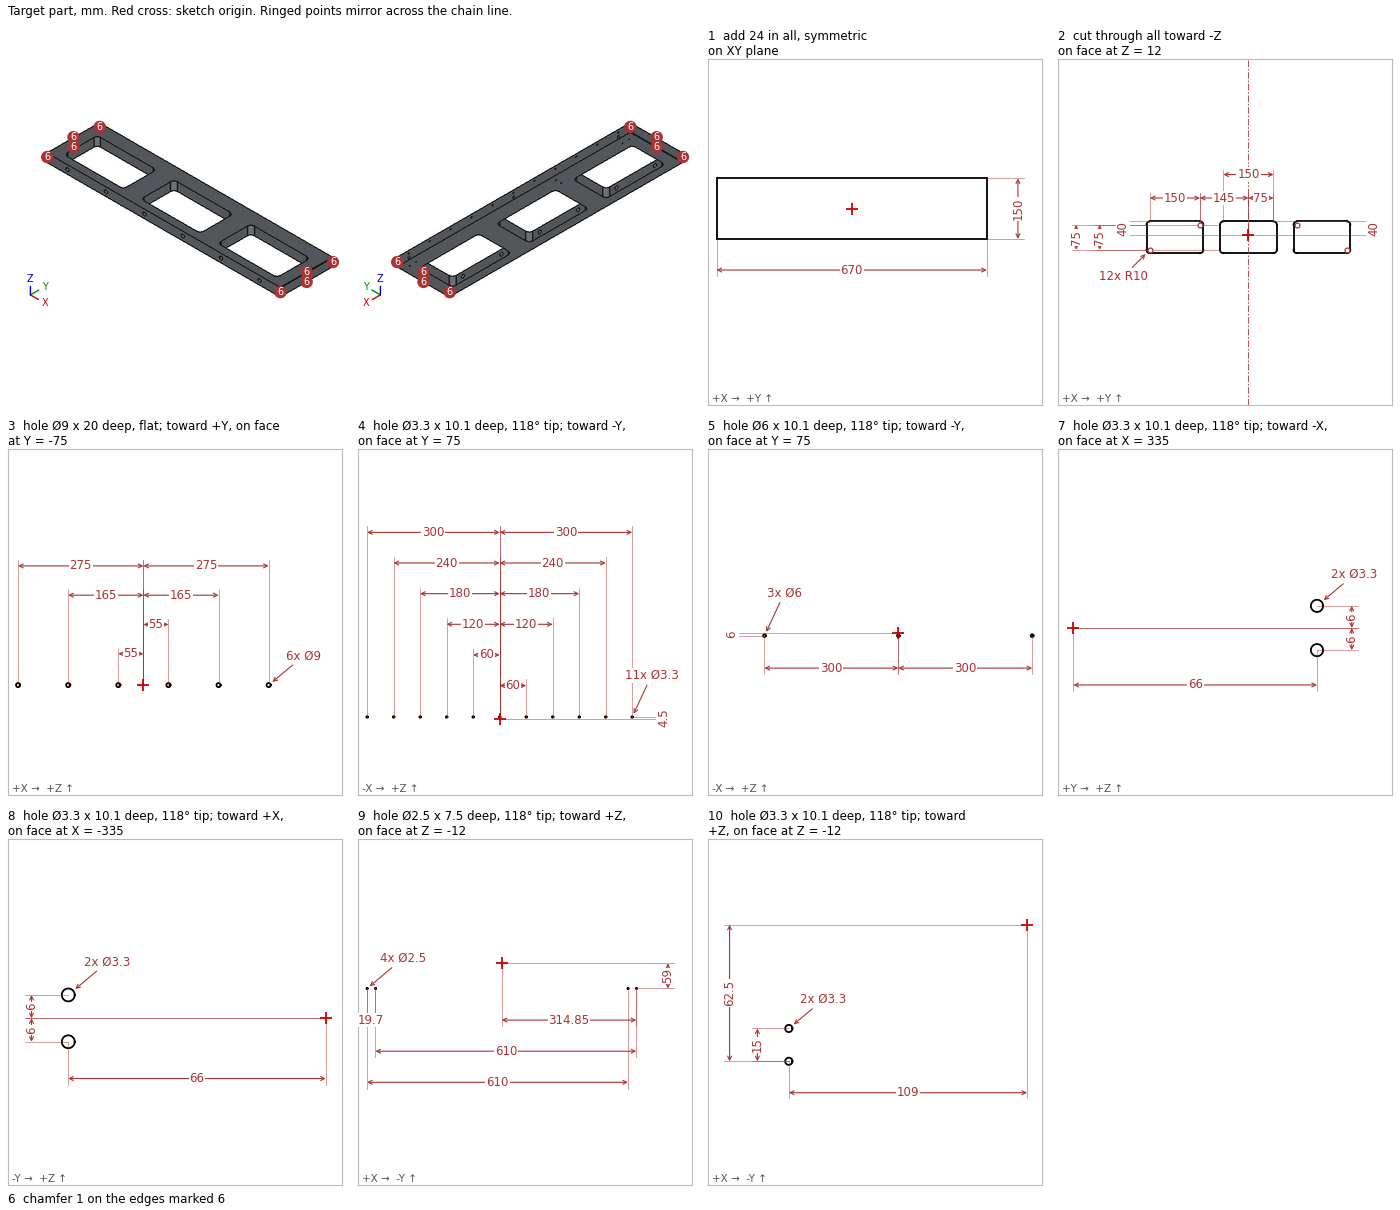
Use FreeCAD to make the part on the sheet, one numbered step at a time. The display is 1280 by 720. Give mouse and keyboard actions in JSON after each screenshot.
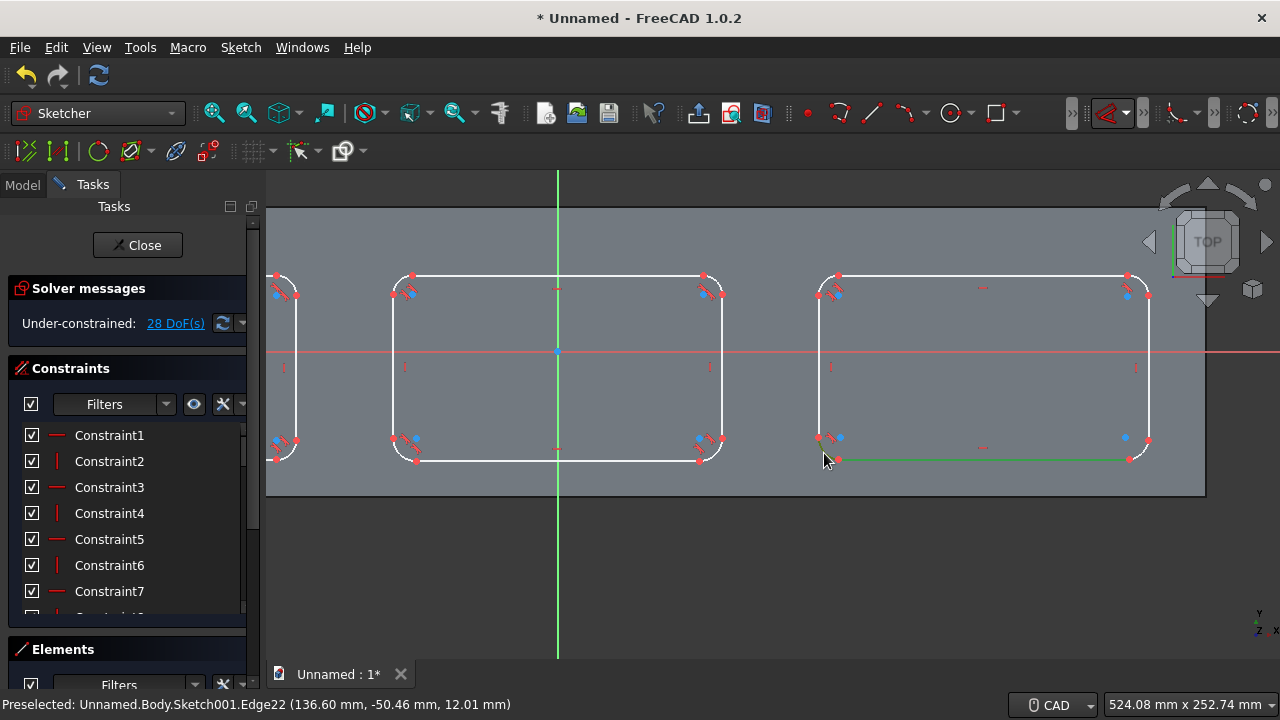
{"action": "key", "text": "t"}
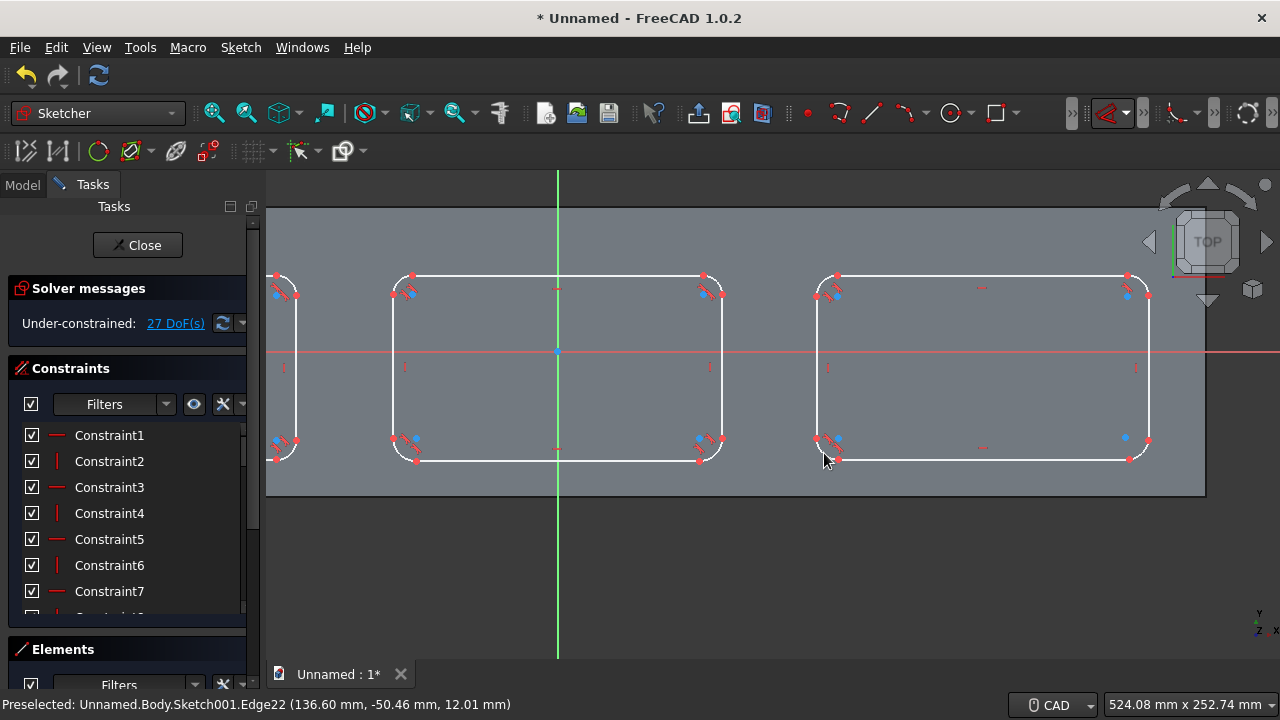
{"action": "left_click", "coordinate": [926, 460]}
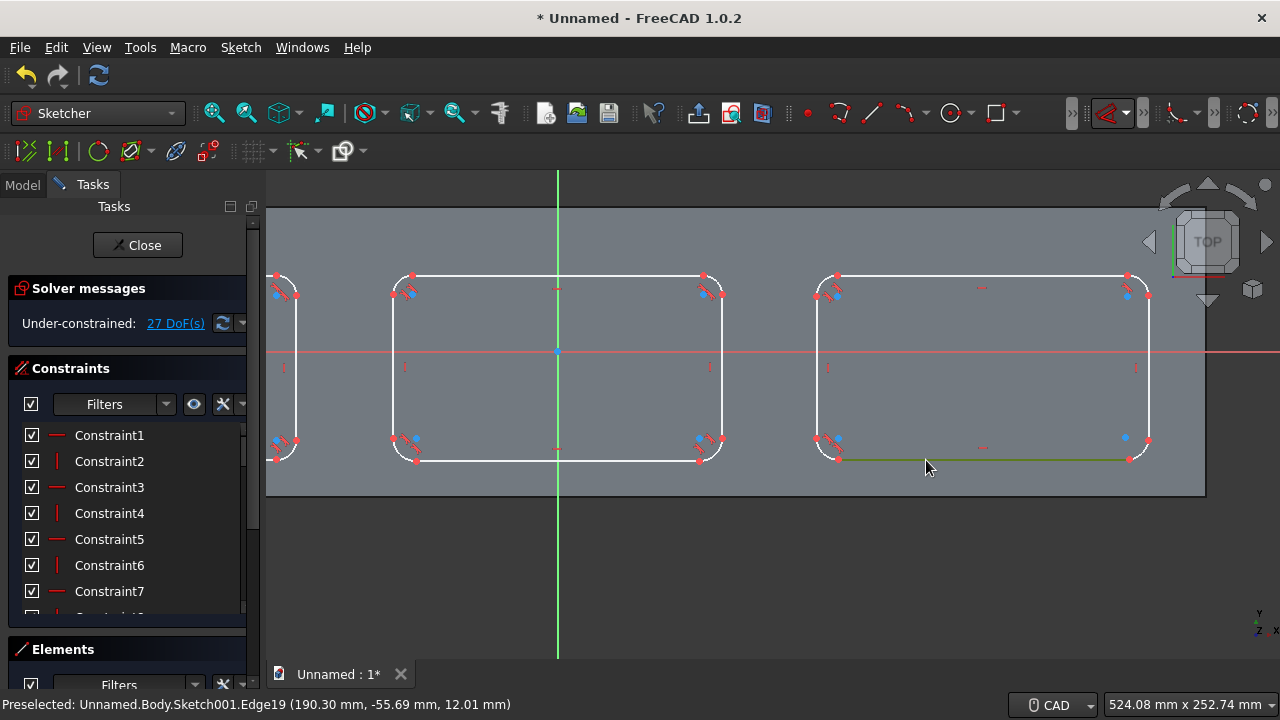
{"action": "scroll", "coordinate": [824, 454], "scroll_direction": "down", "scroll_amount": 4}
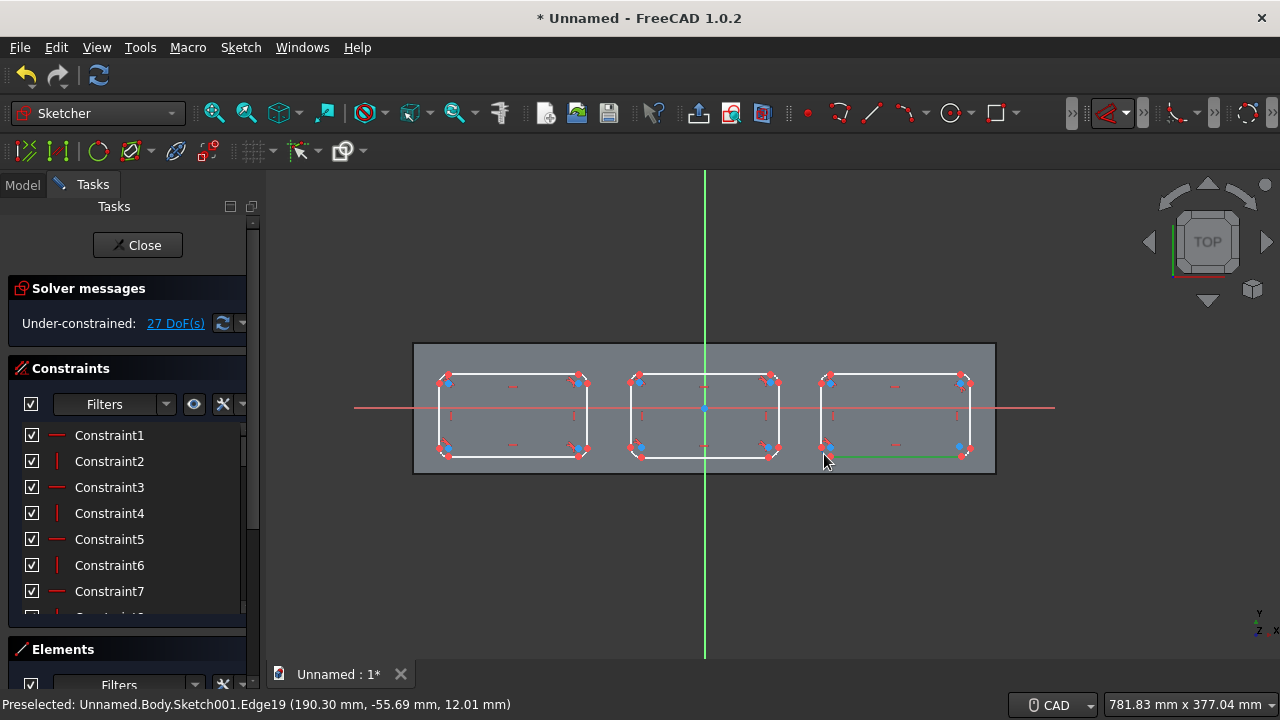
{"action": "scroll", "coordinate": [967, 454], "scroll_direction": "up", "scroll_amount": 4}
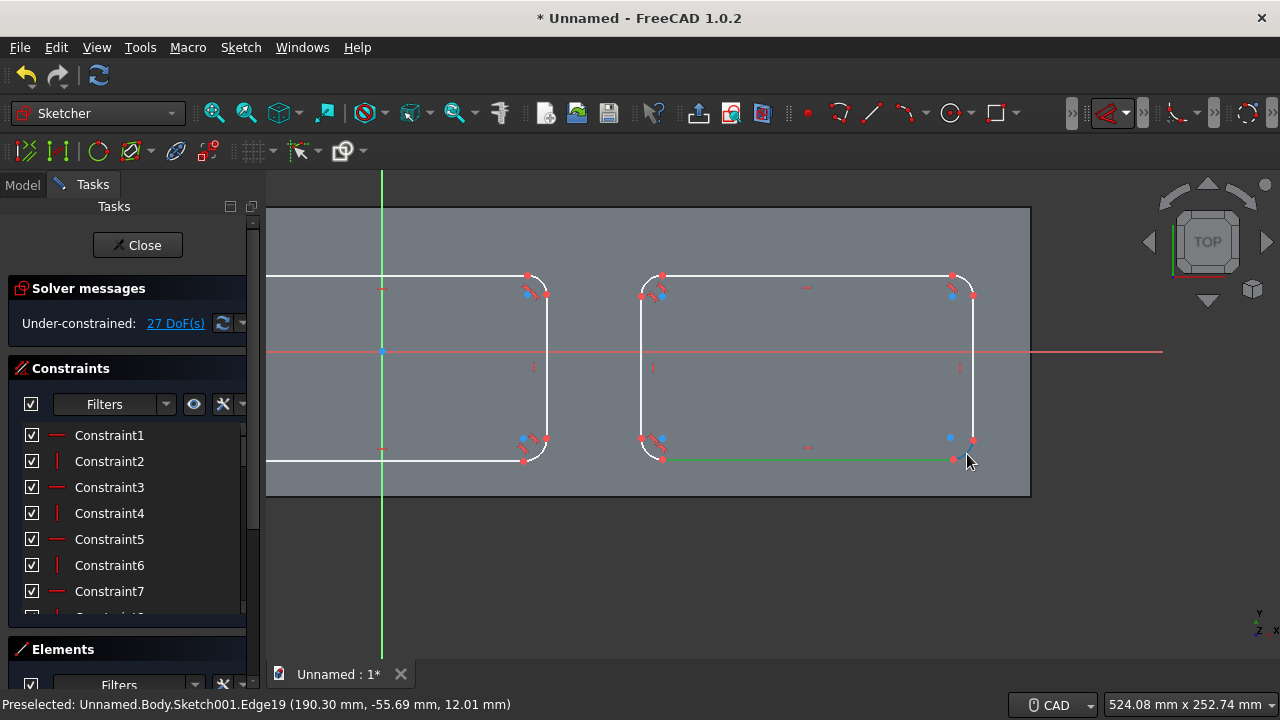
{"action": "left_click", "coordinate": [967, 453]}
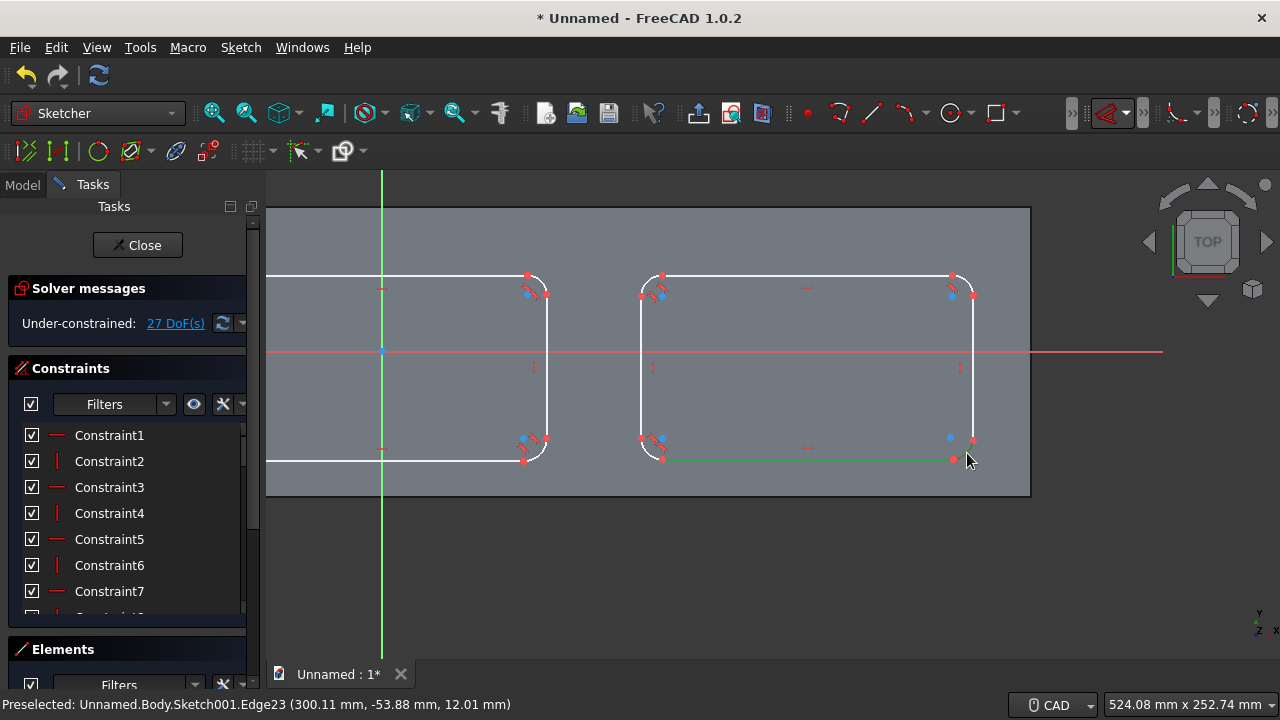
{"action": "key", "text": "t"}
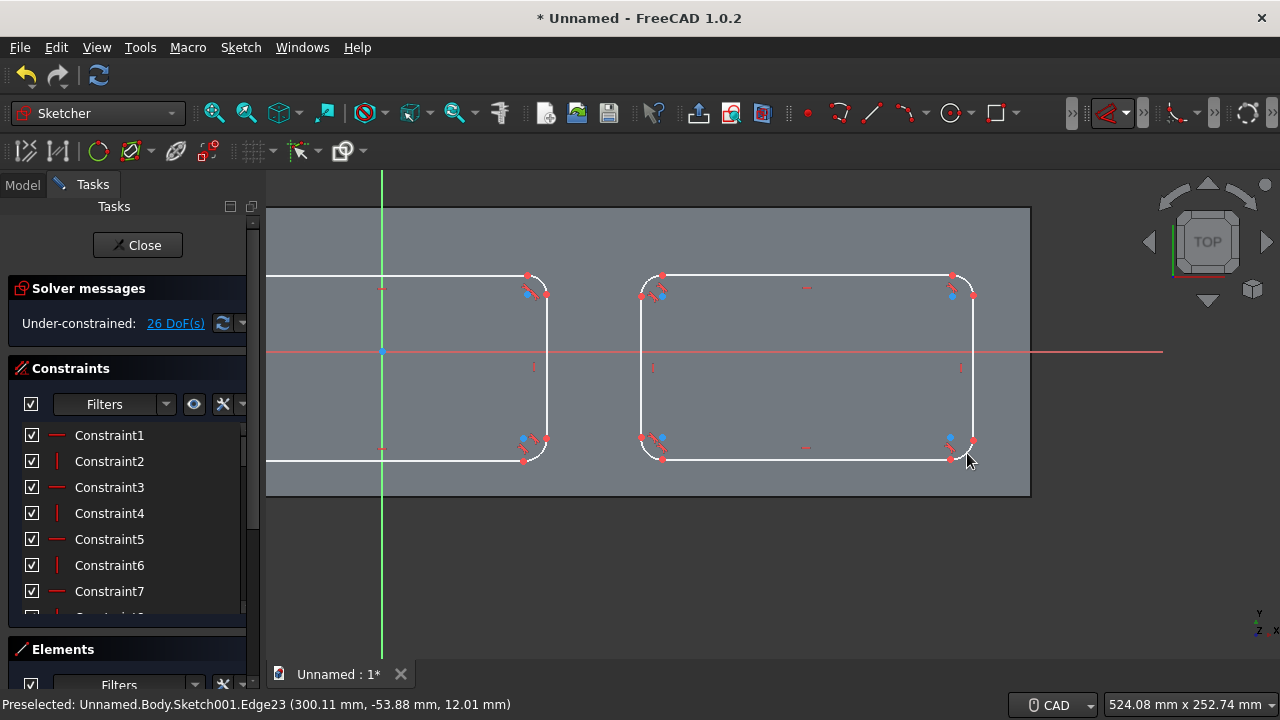
{"action": "left_click", "coordinate": [973, 397]}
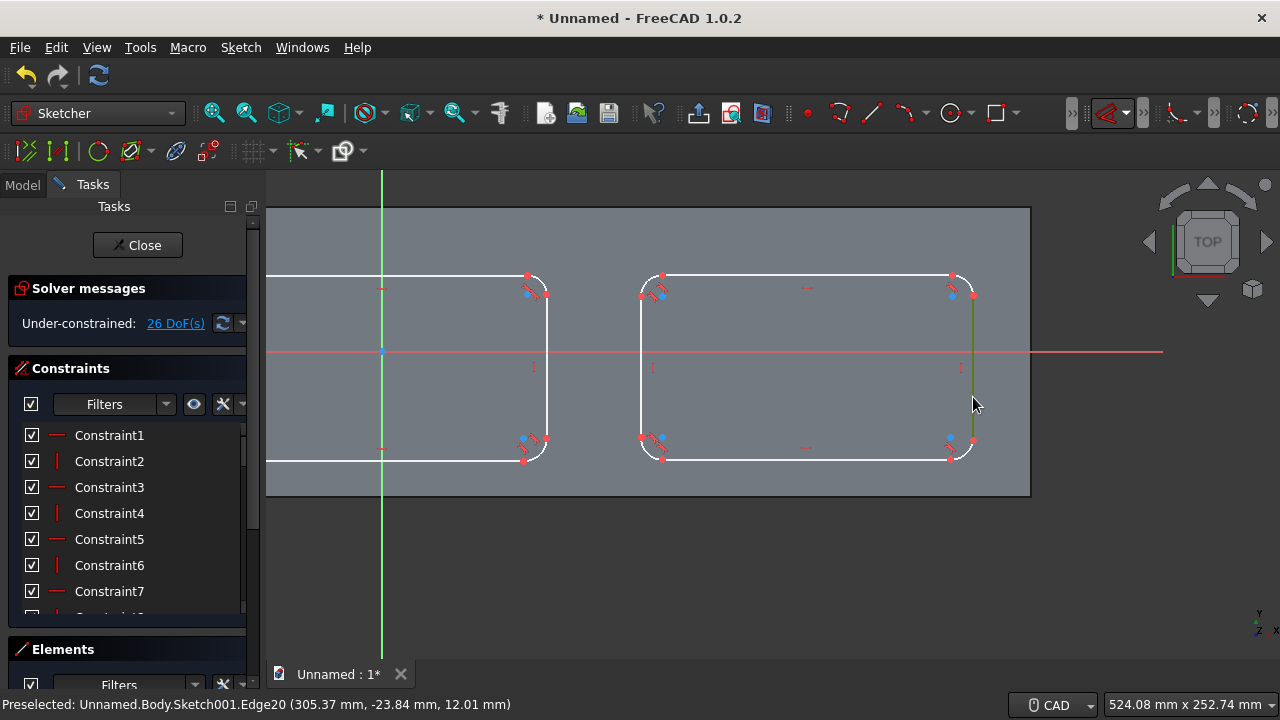
{"action": "scroll", "coordinate": [960, 458], "scroll_direction": "up", "scroll_amount": 2}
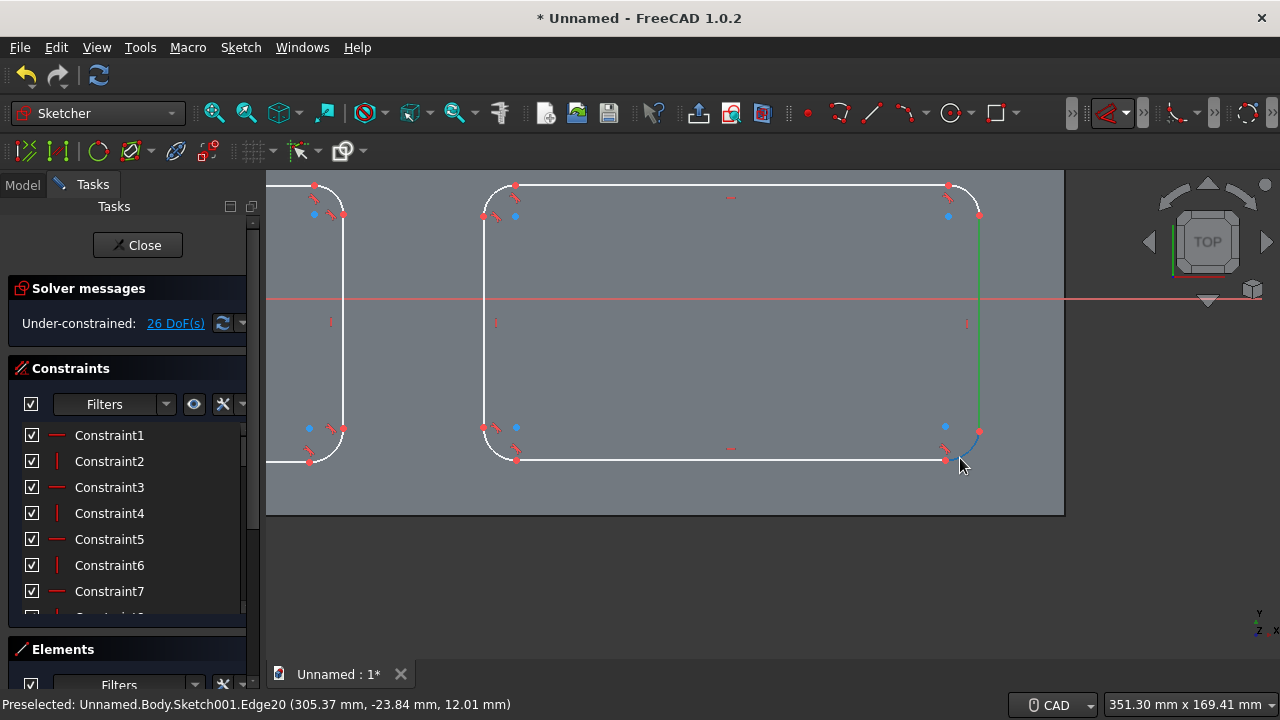
{"action": "left_click", "coordinate": [960, 457]}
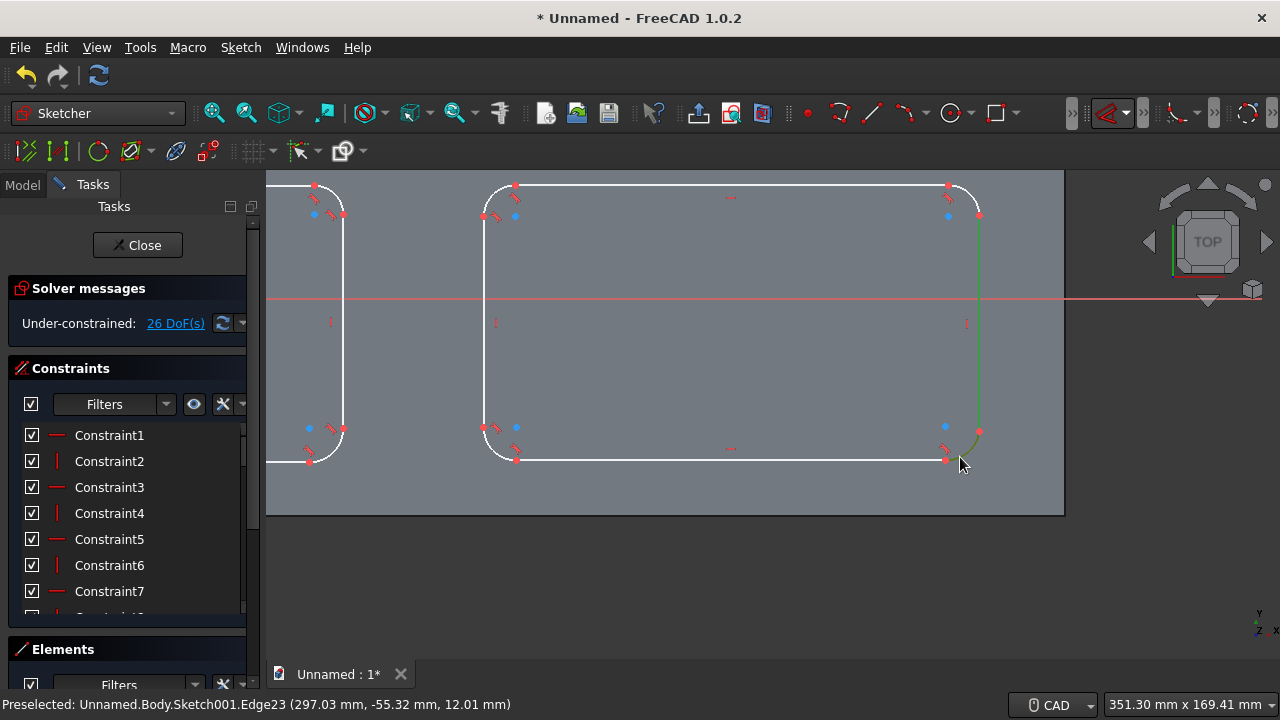
{"action": "key", "text": "t"}